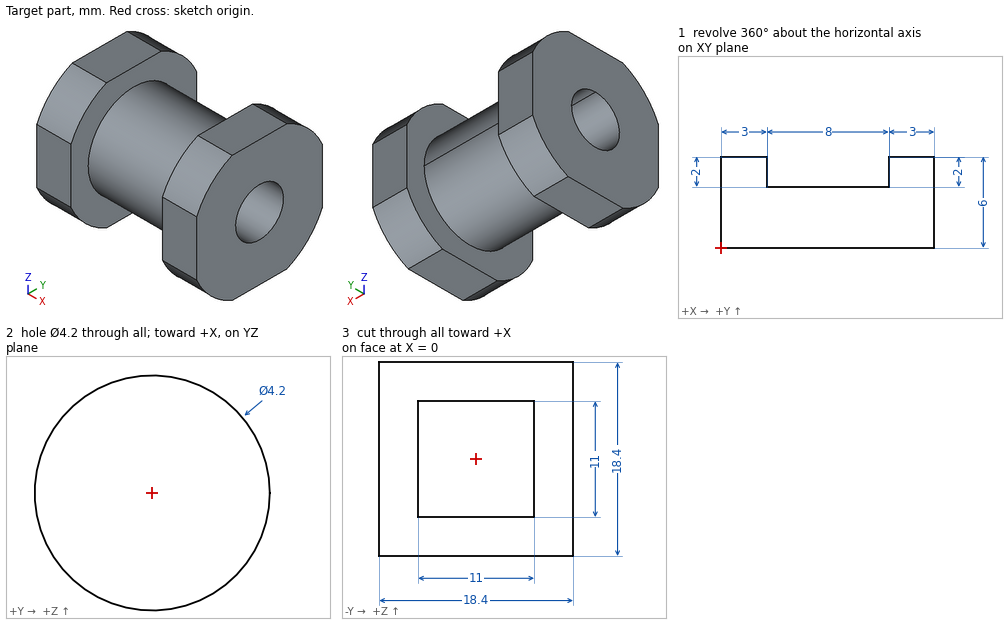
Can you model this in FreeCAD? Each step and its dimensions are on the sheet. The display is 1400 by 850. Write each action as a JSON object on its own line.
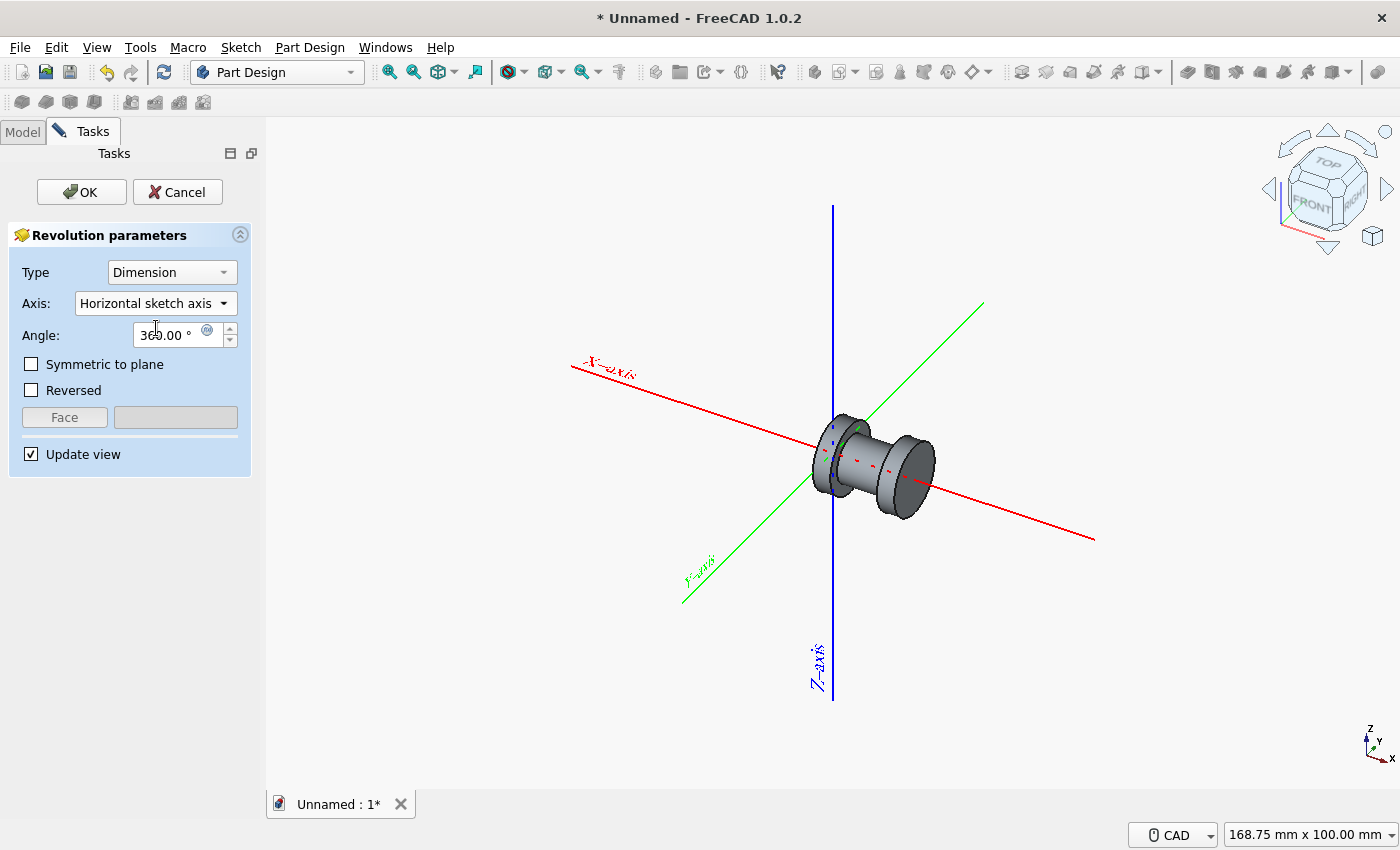
{"action": "left_click", "coordinate": [82, 192]}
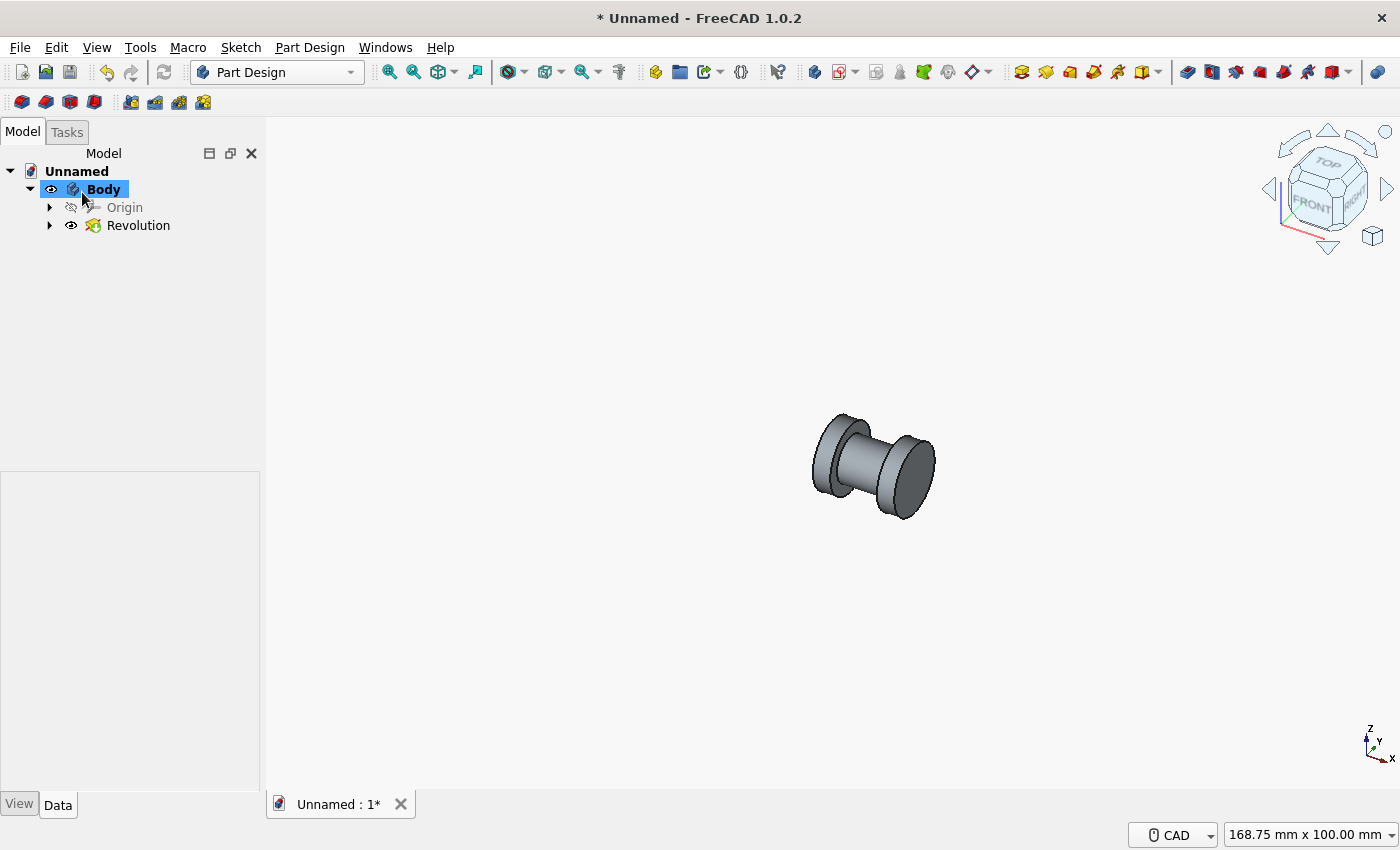
{"action": "left_click", "coordinate": [390, 72]}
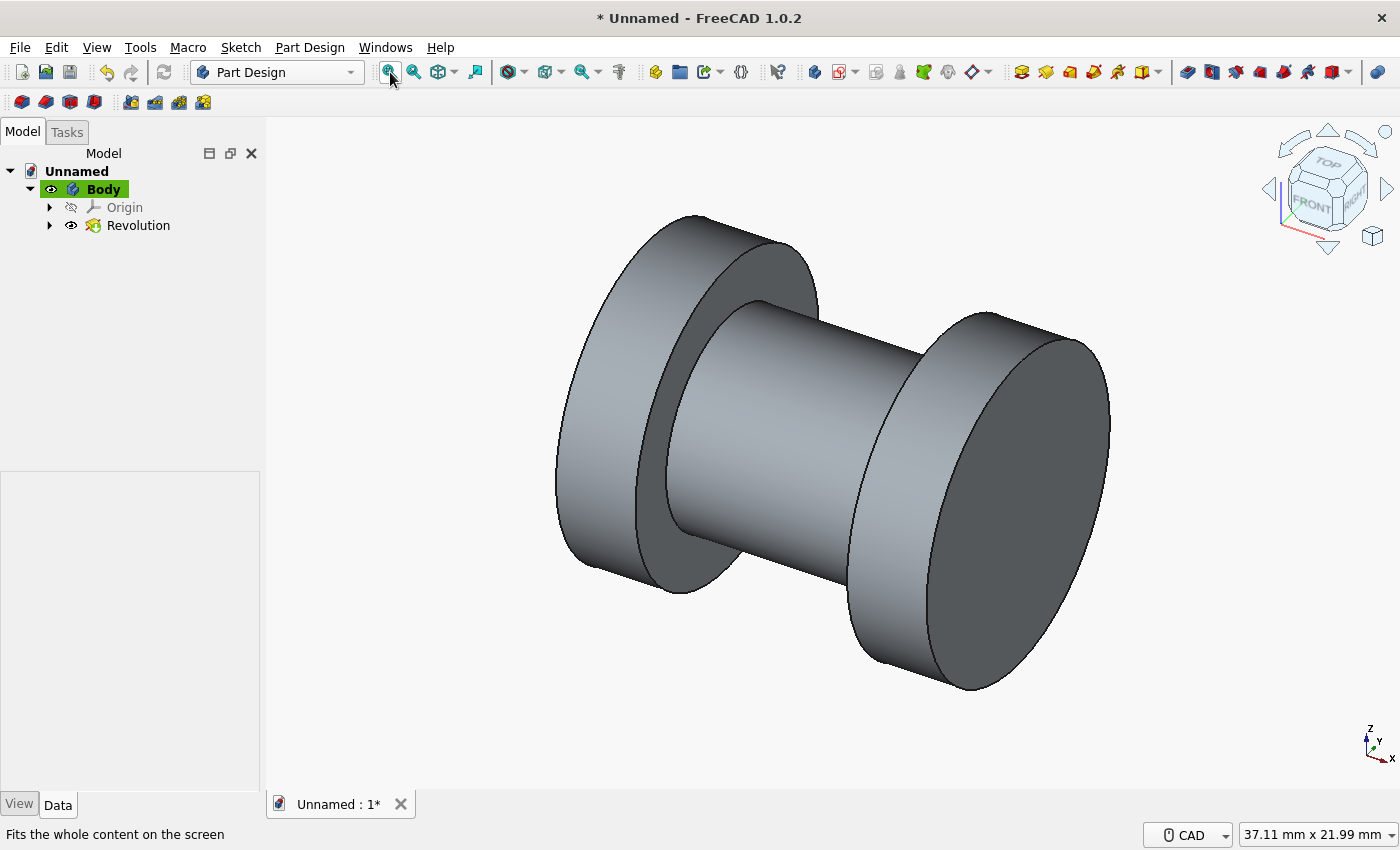
{"action": "left_click", "coordinate": [840, 72]}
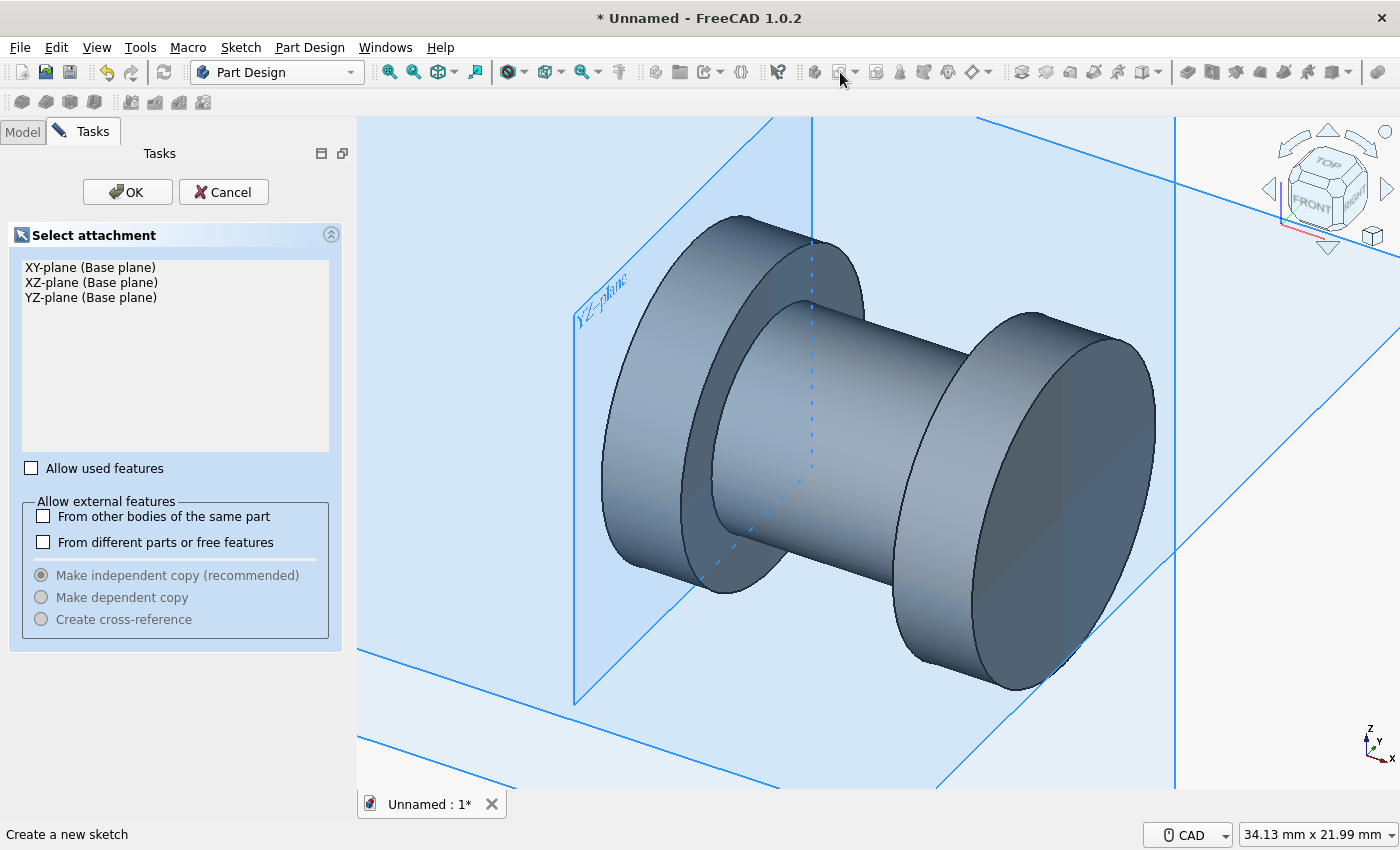
{"action": "left_click", "coordinate": [82, 298]}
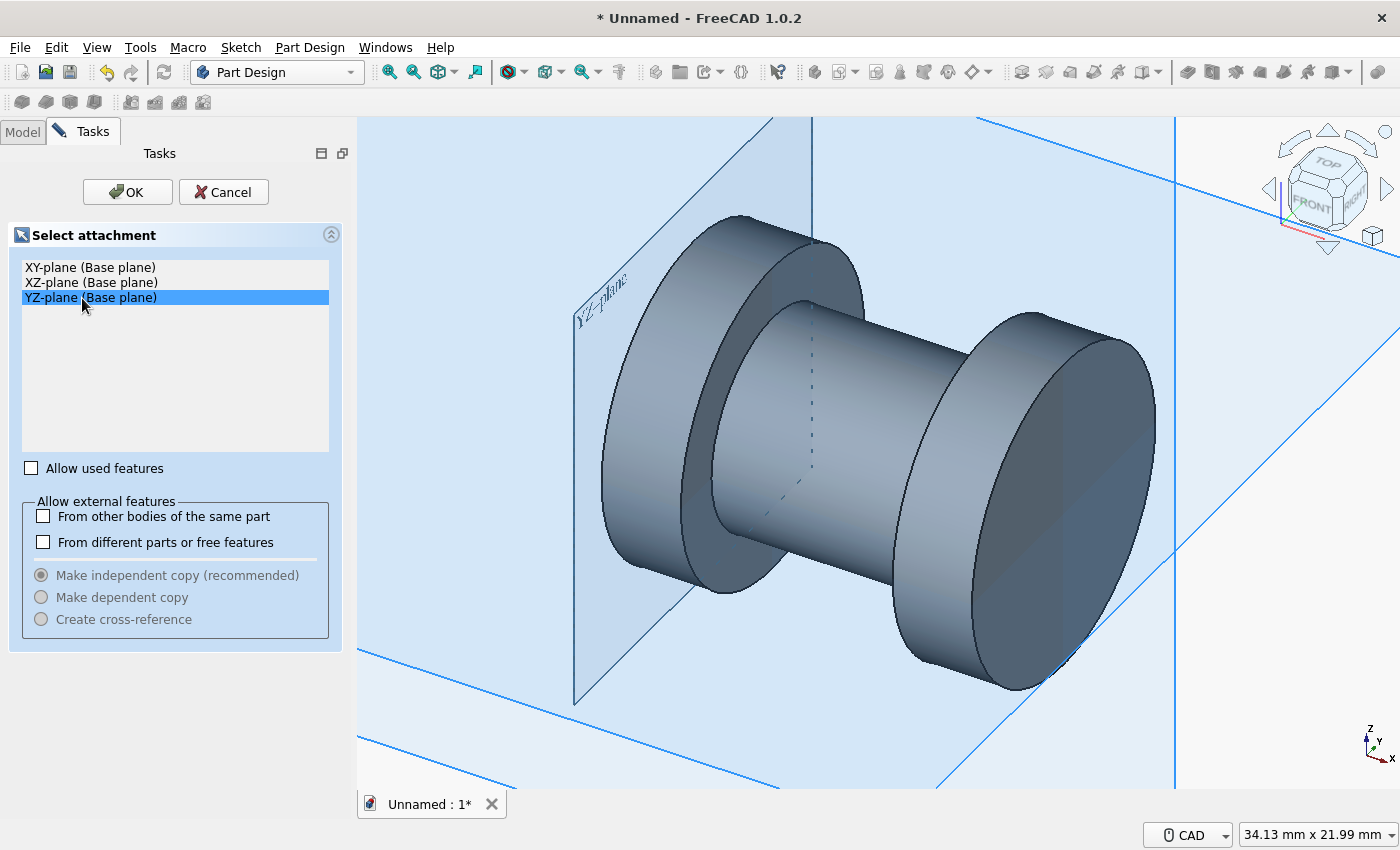
{"action": "left_click", "coordinate": [128, 192]}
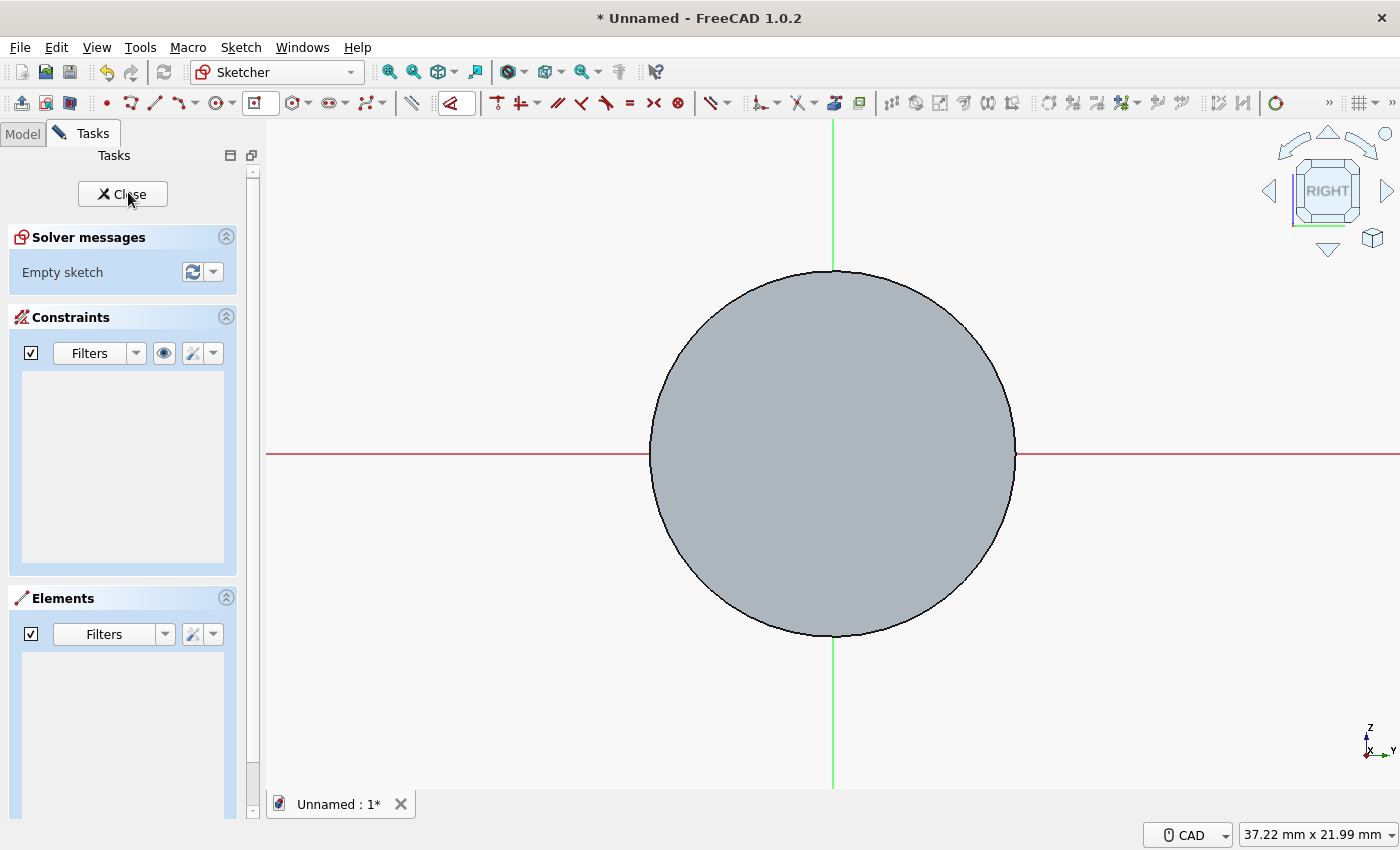
{"action": "left_click", "coordinate": [70, 104]}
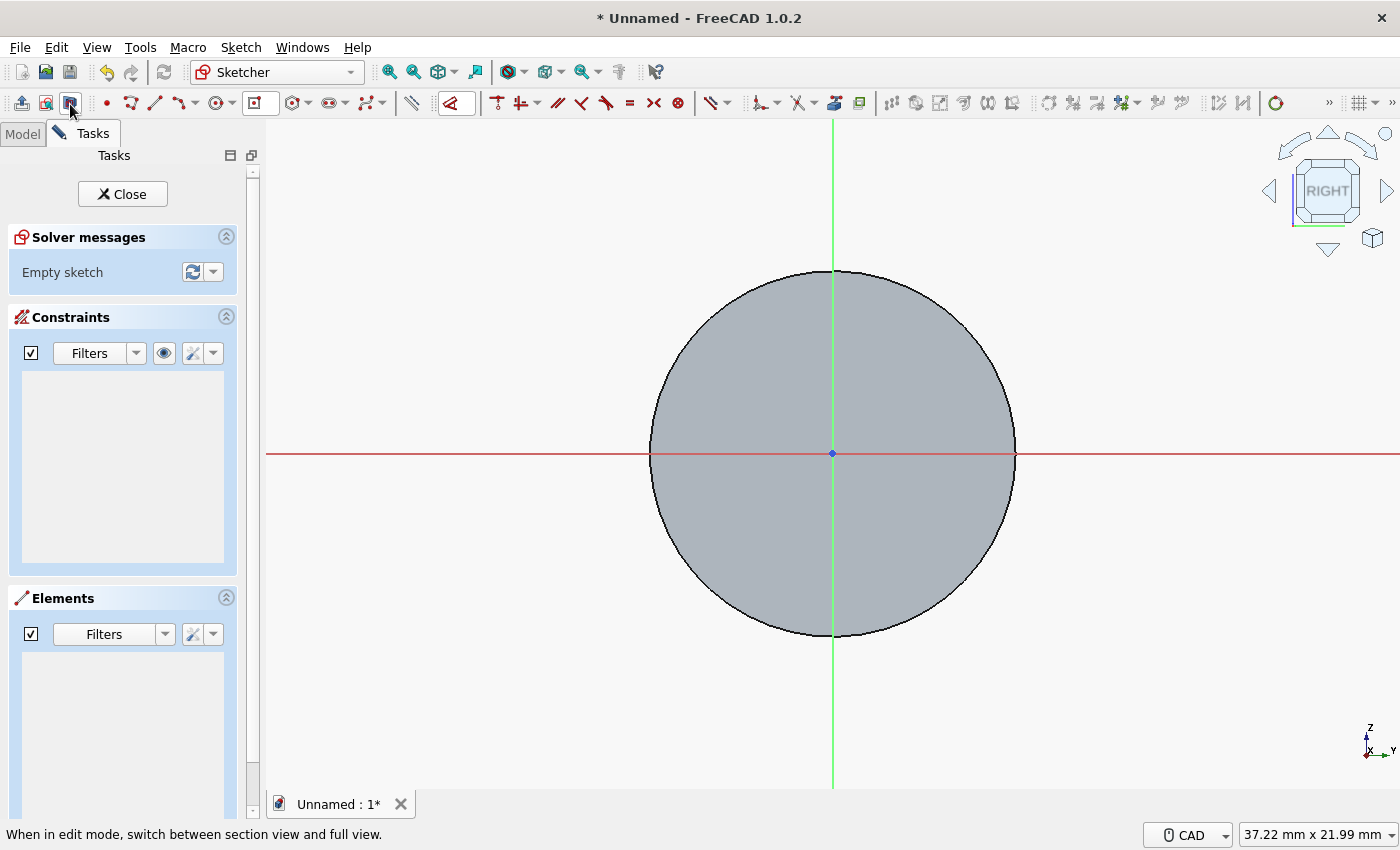
{"action": "scroll", "coordinate": [862, 454], "scroll_direction": "up", "scroll_amount": 6}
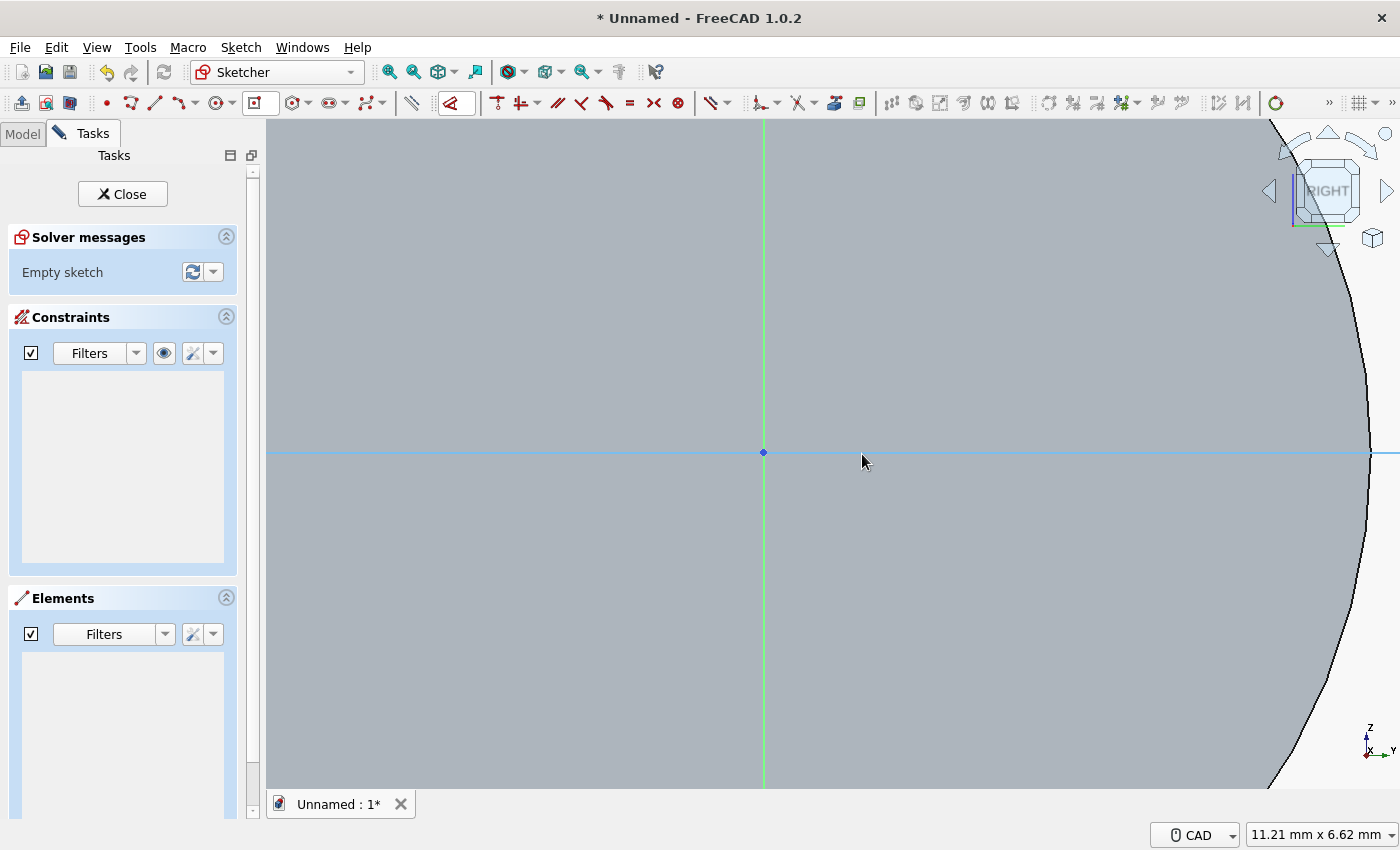
{"action": "left_click", "coordinate": [216, 104]}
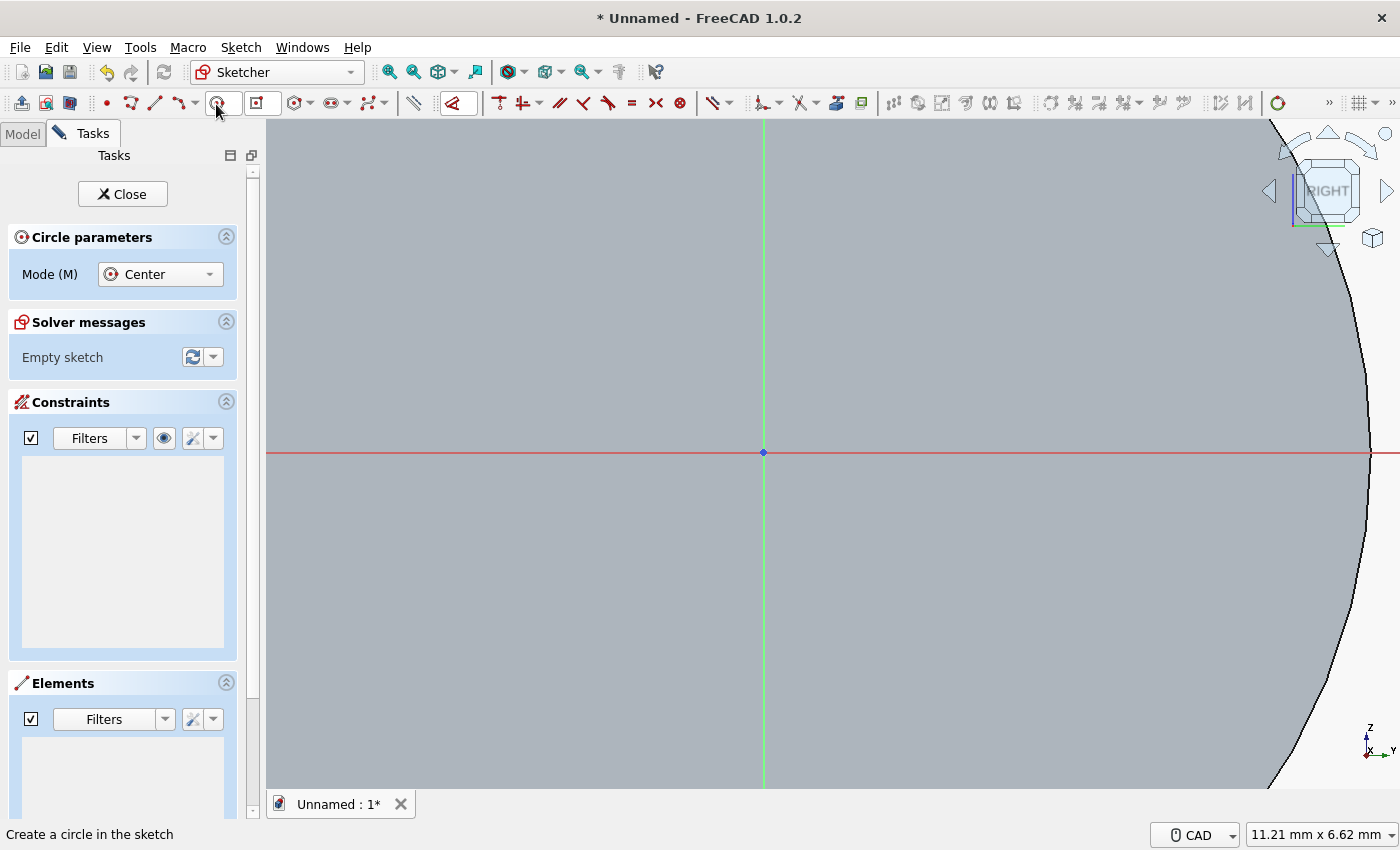
{"action": "left_click", "coordinate": [764, 453]}
{"action": "mouse_move", "coordinate": [914, 303]}